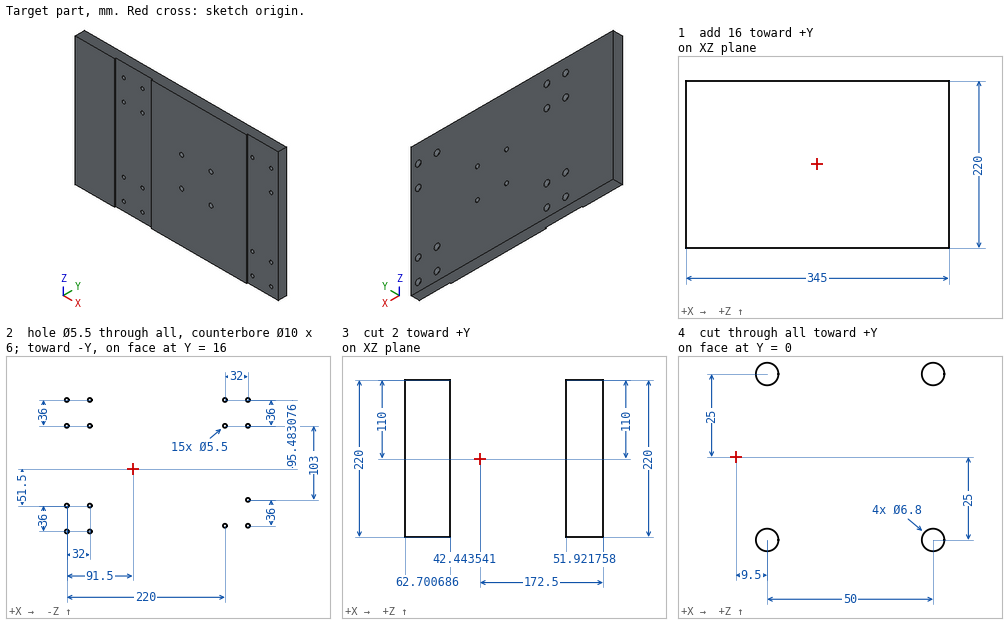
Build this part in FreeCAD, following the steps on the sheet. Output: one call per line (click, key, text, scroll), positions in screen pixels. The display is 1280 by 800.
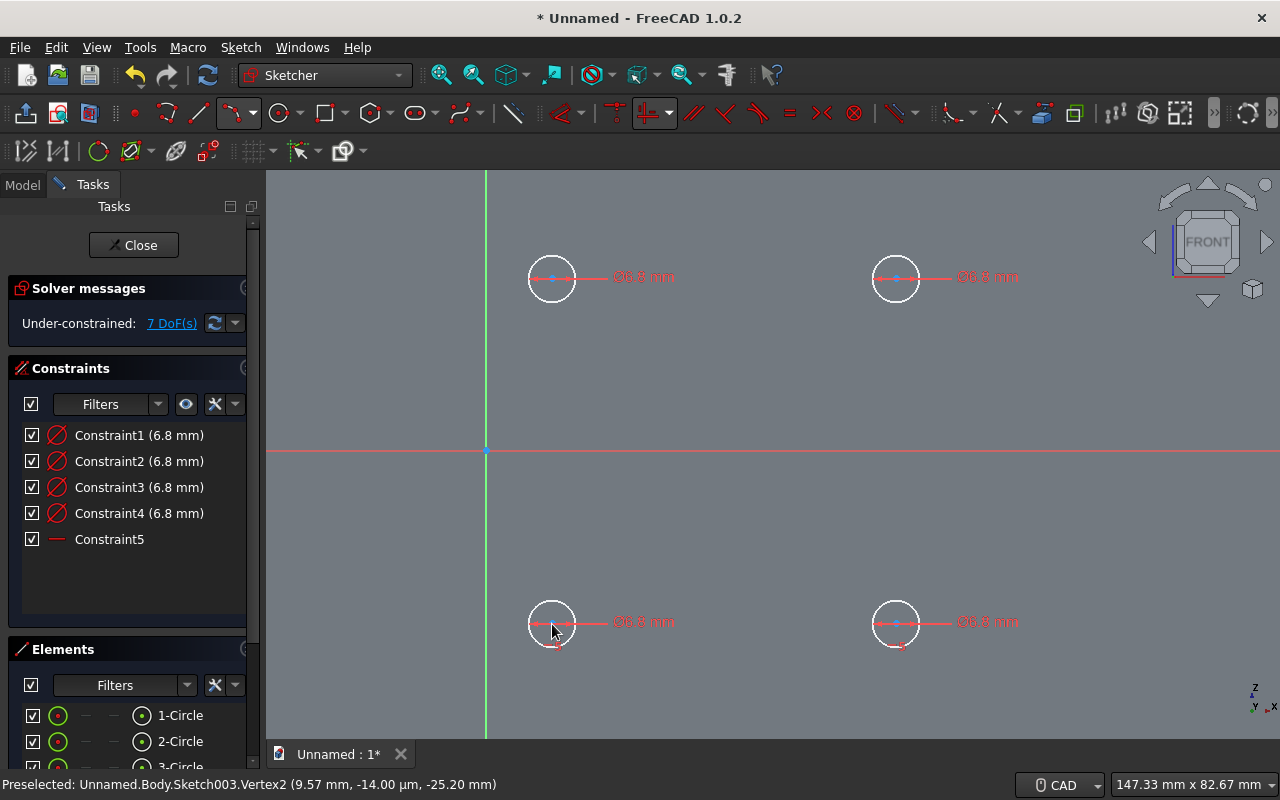
click(552, 624)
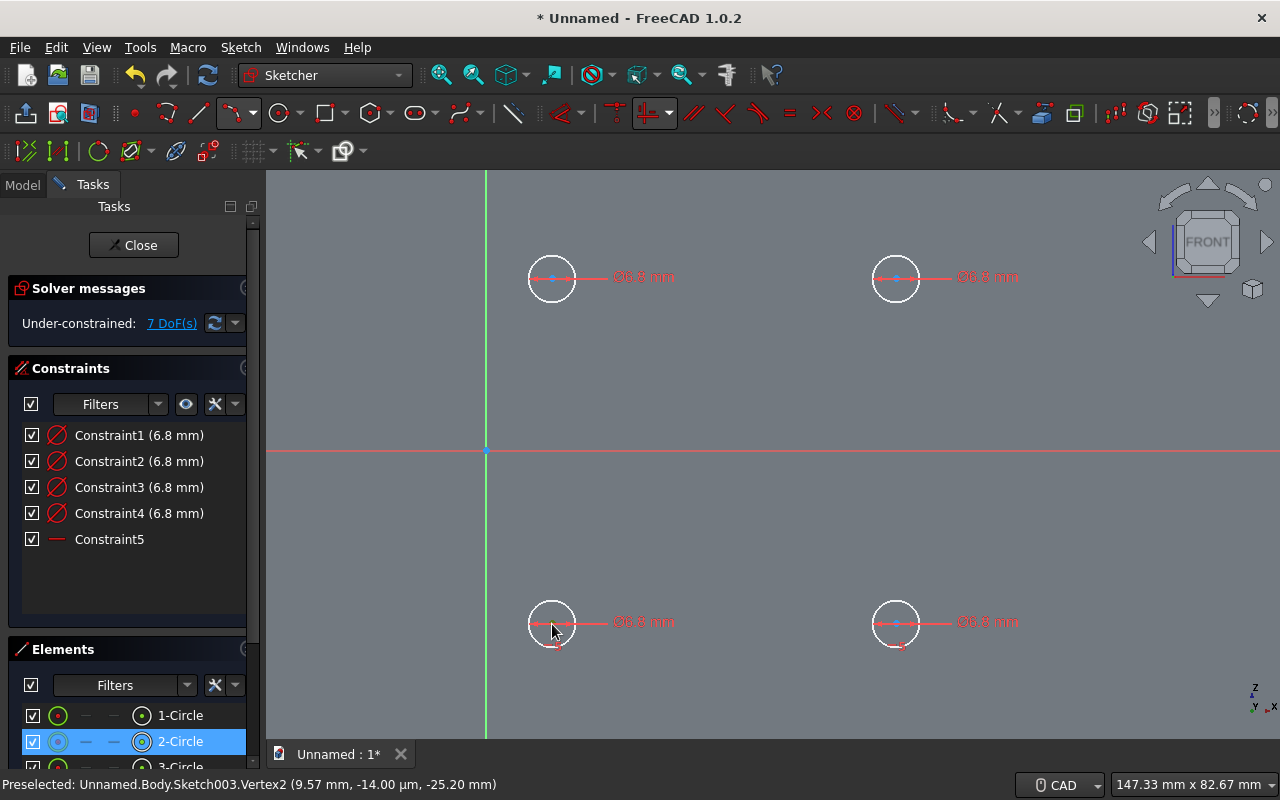
click(552, 279)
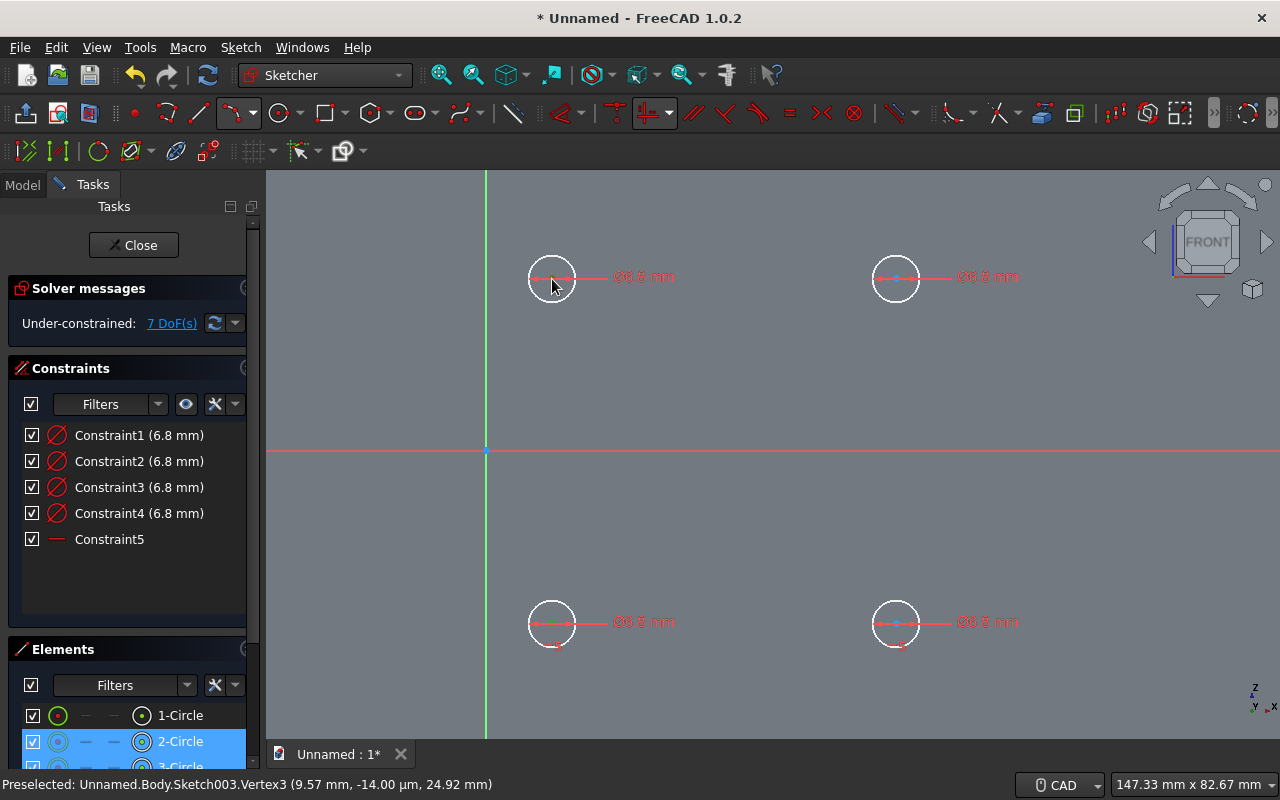
click(672, 114)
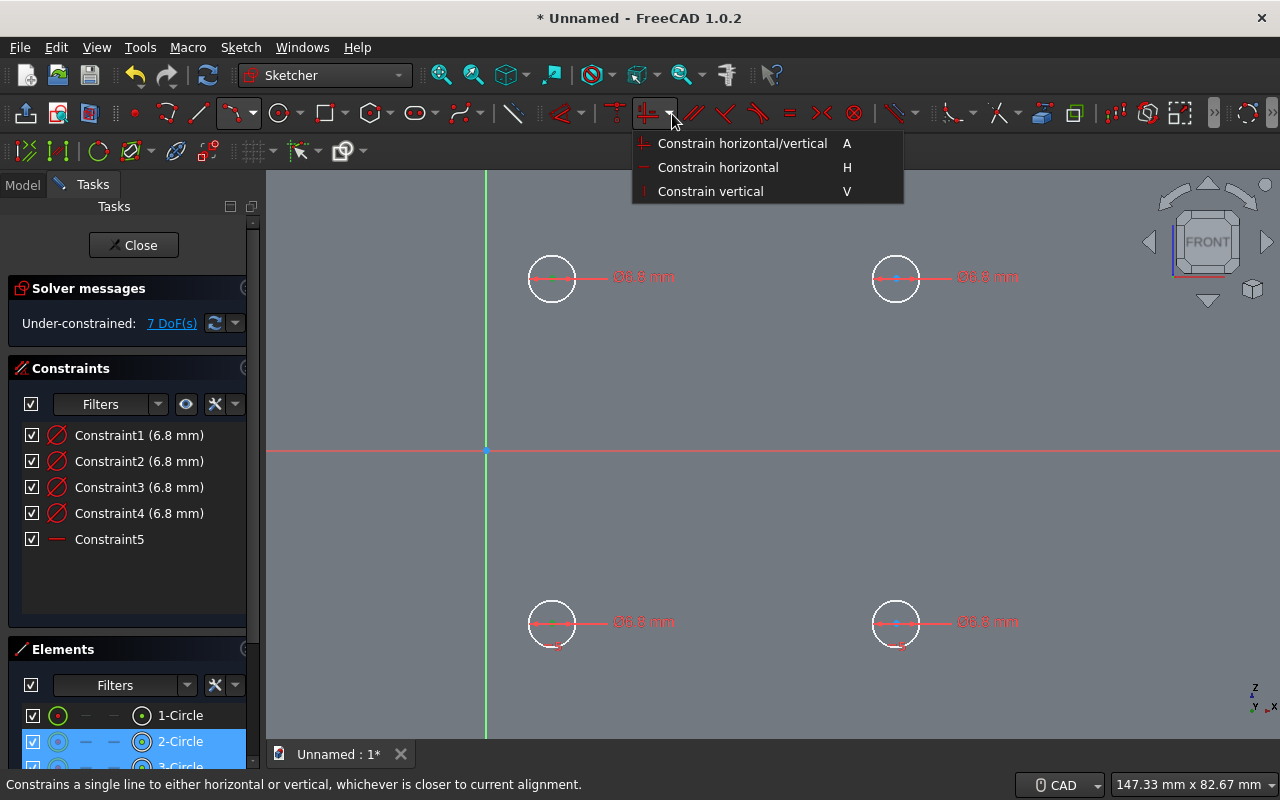
click(768, 191)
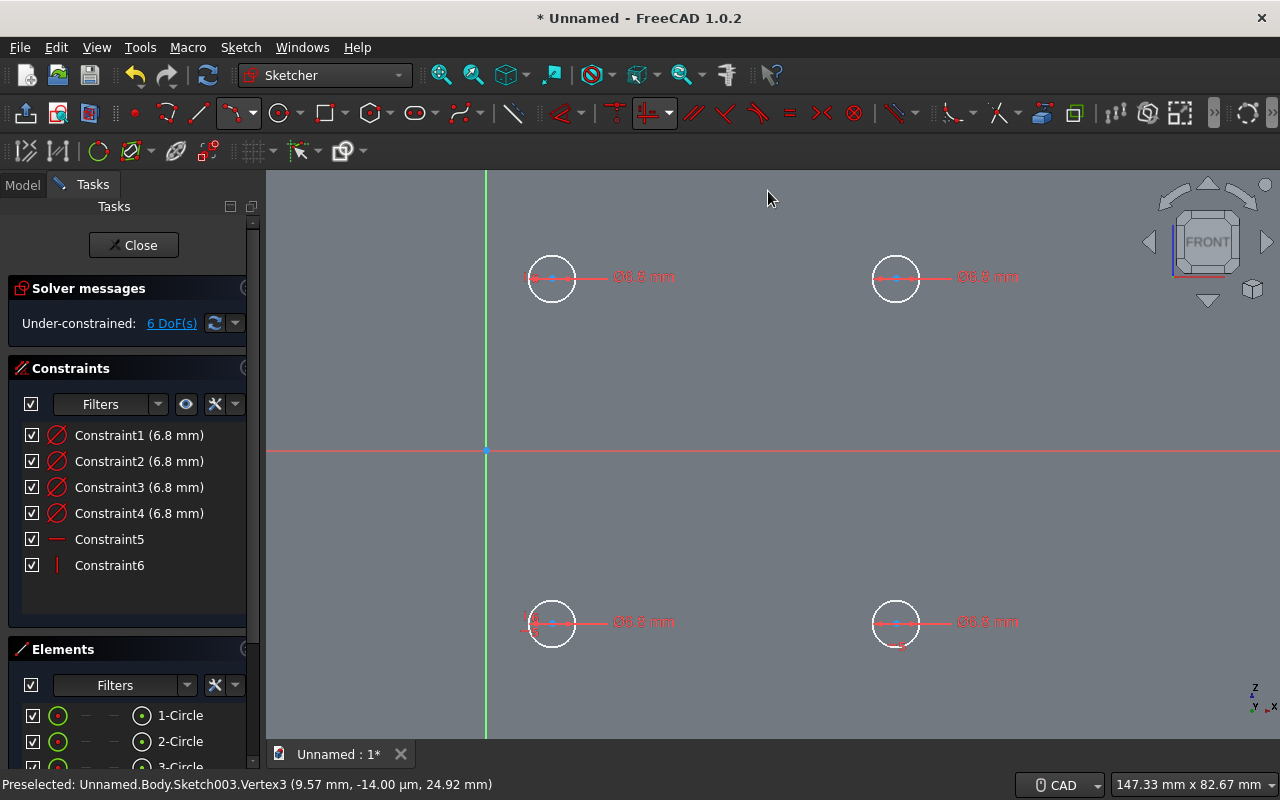
click(896, 624)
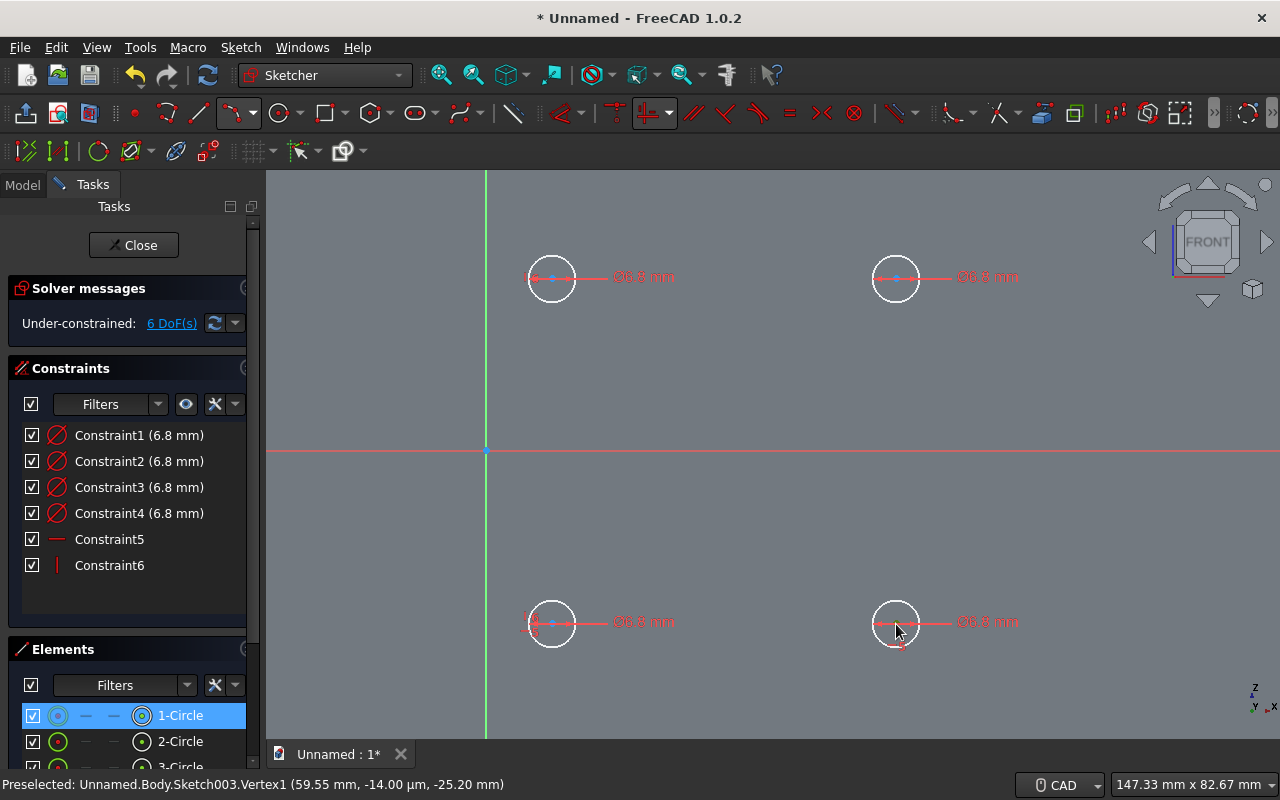
click(896, 279)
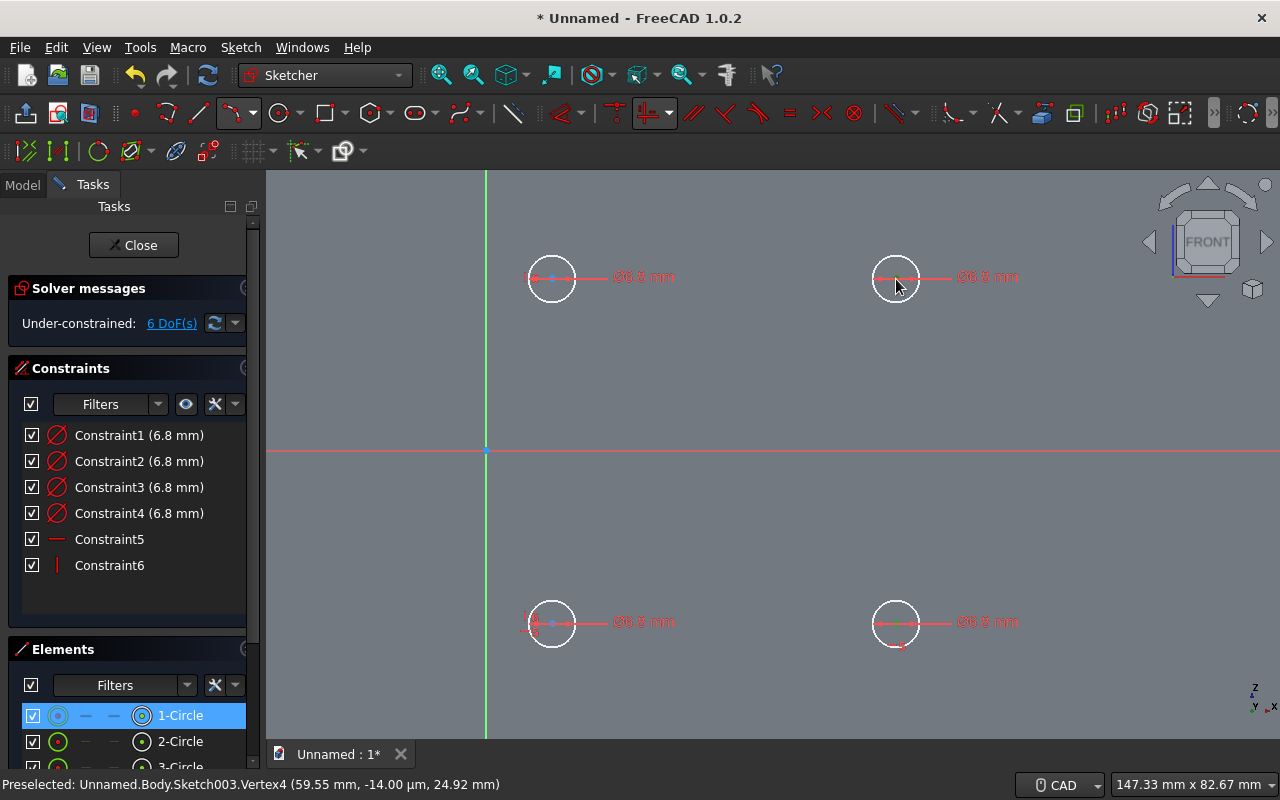
key(v)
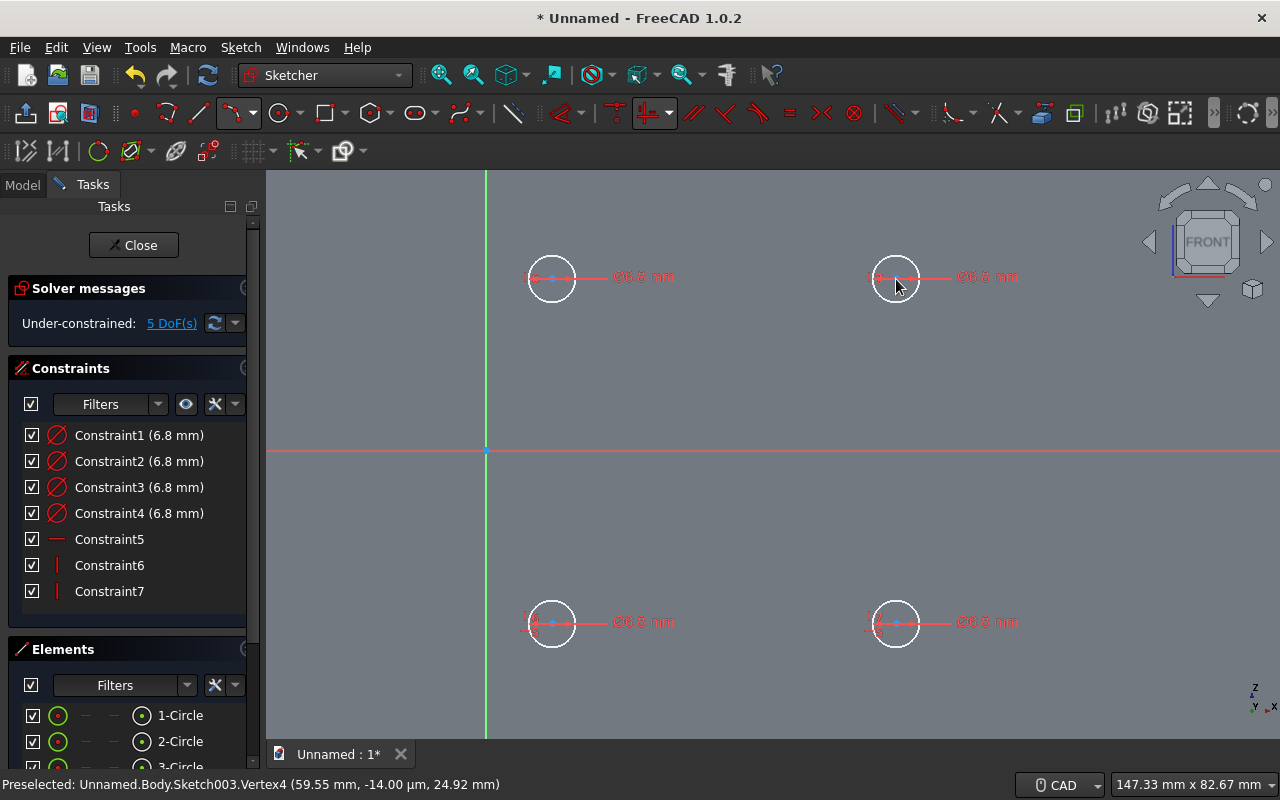
click(552, 279)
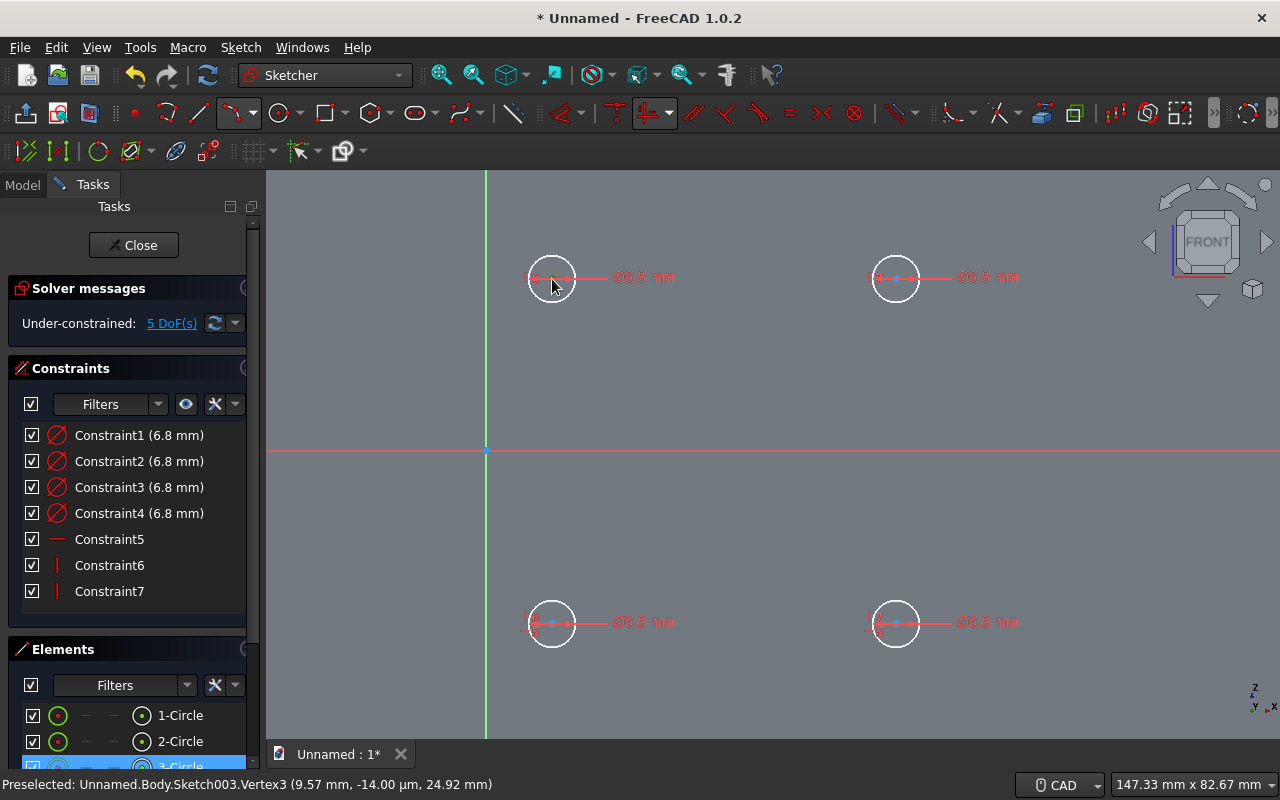
click(896, 279)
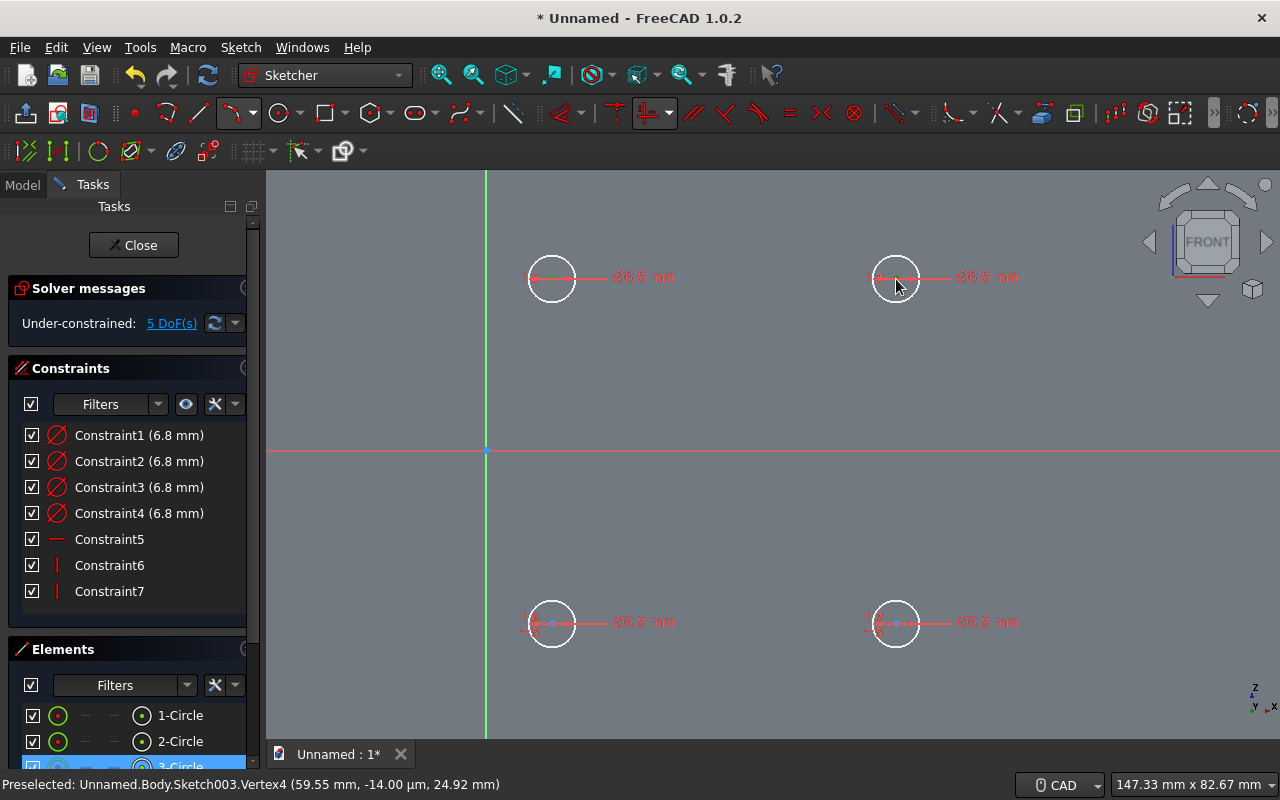
click(672, 114)